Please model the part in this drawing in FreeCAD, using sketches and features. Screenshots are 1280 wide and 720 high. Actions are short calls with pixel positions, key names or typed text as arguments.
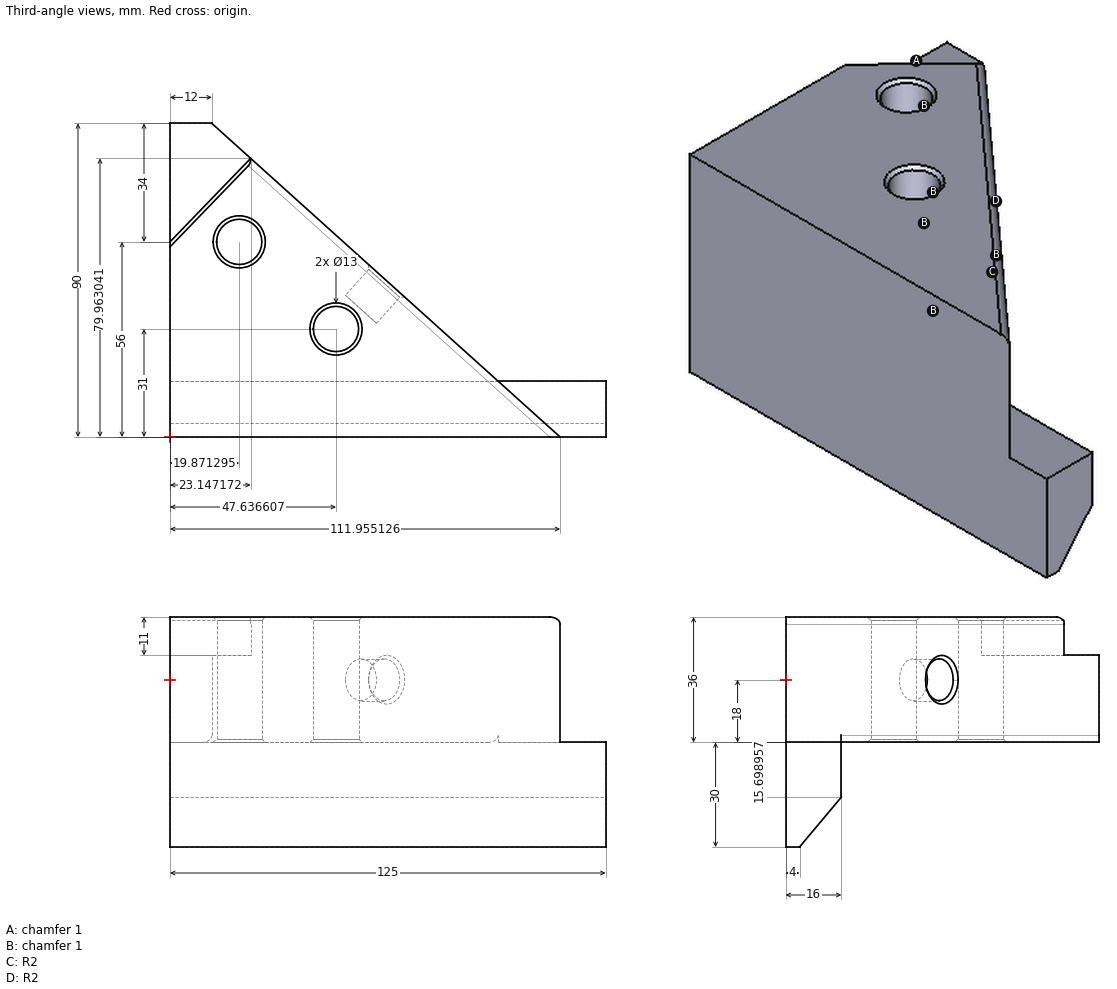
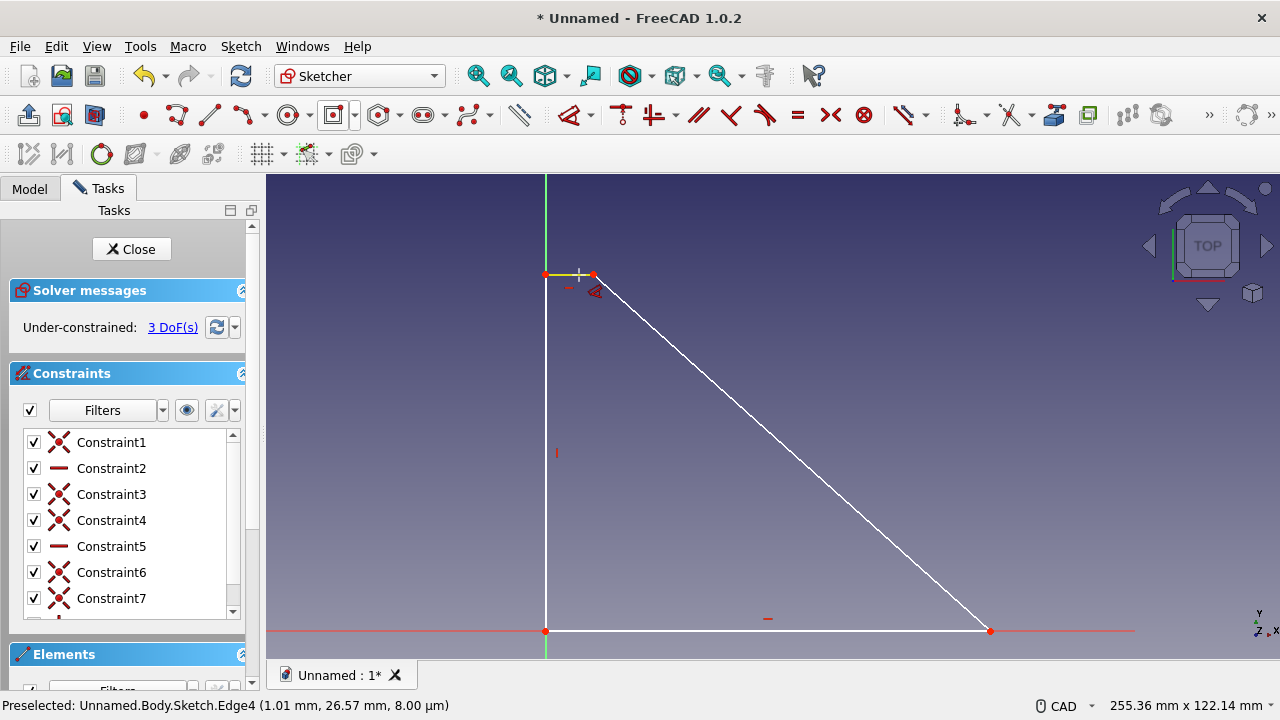
click(579, 275)
click(570, 241)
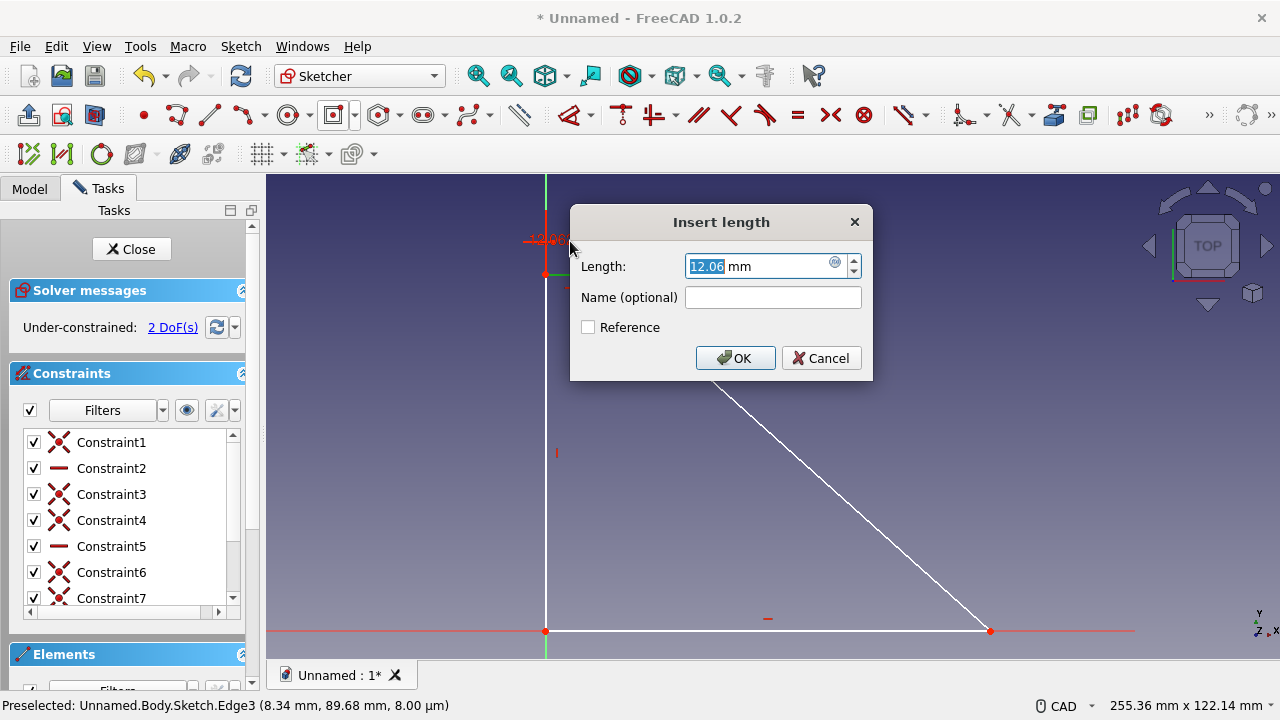
text(12)
key(Return)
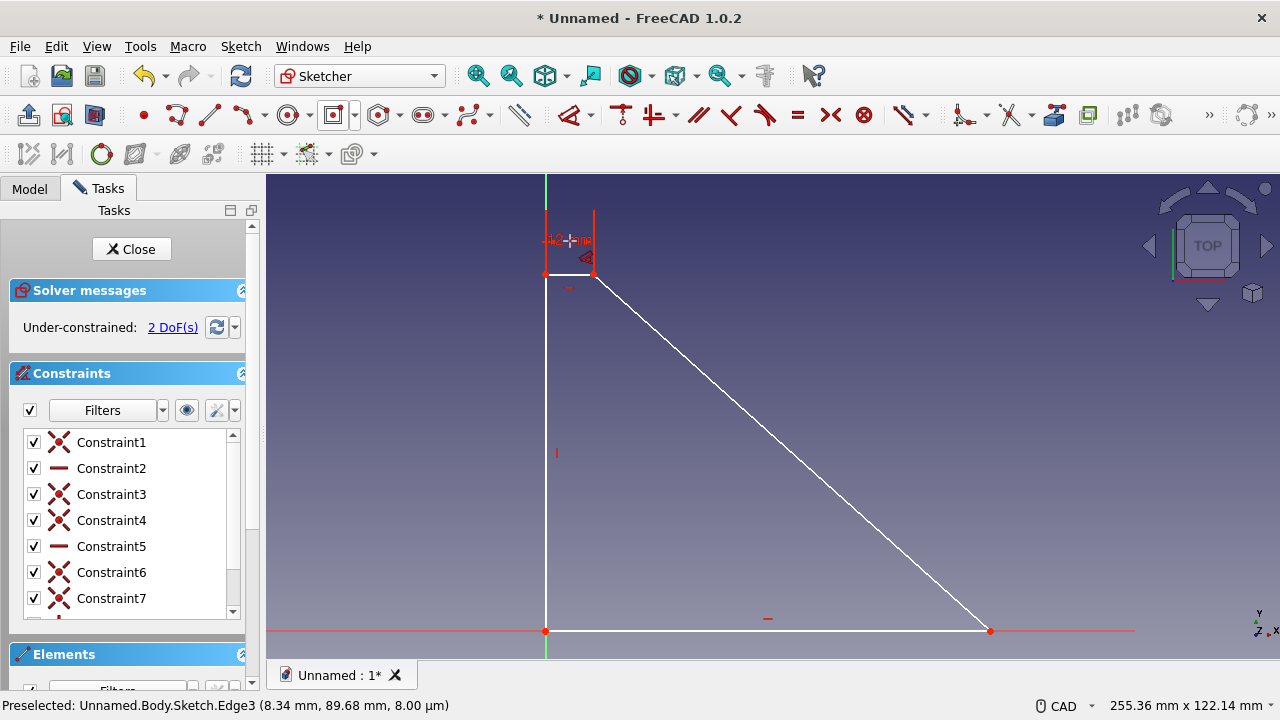
click(546, 382)
click(512, 453)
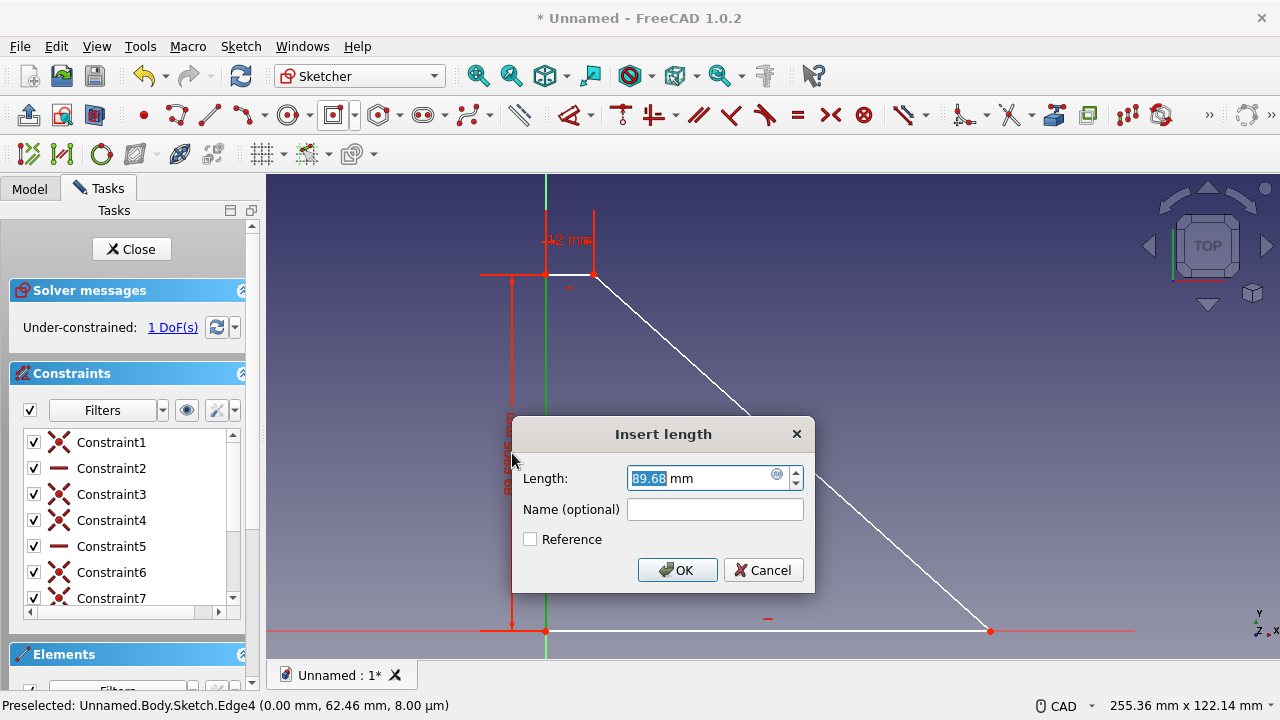
text(90)
key(Return)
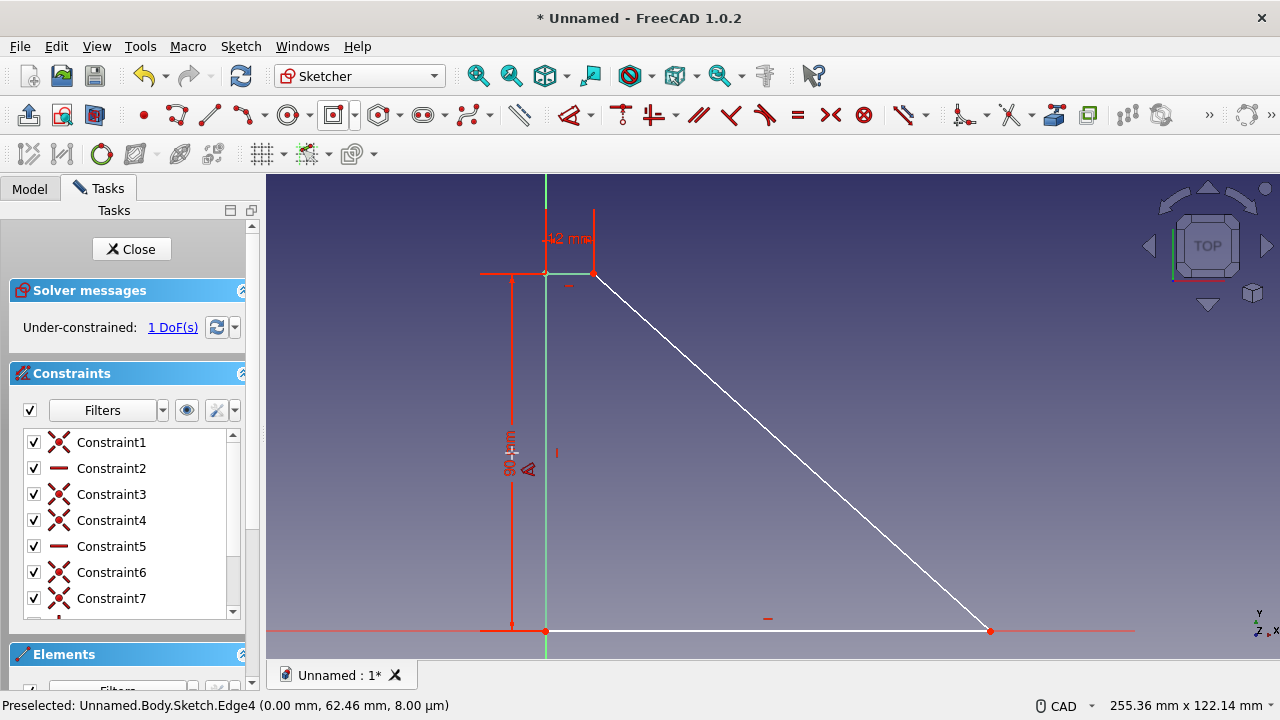
scroll(417, 255, down, 1)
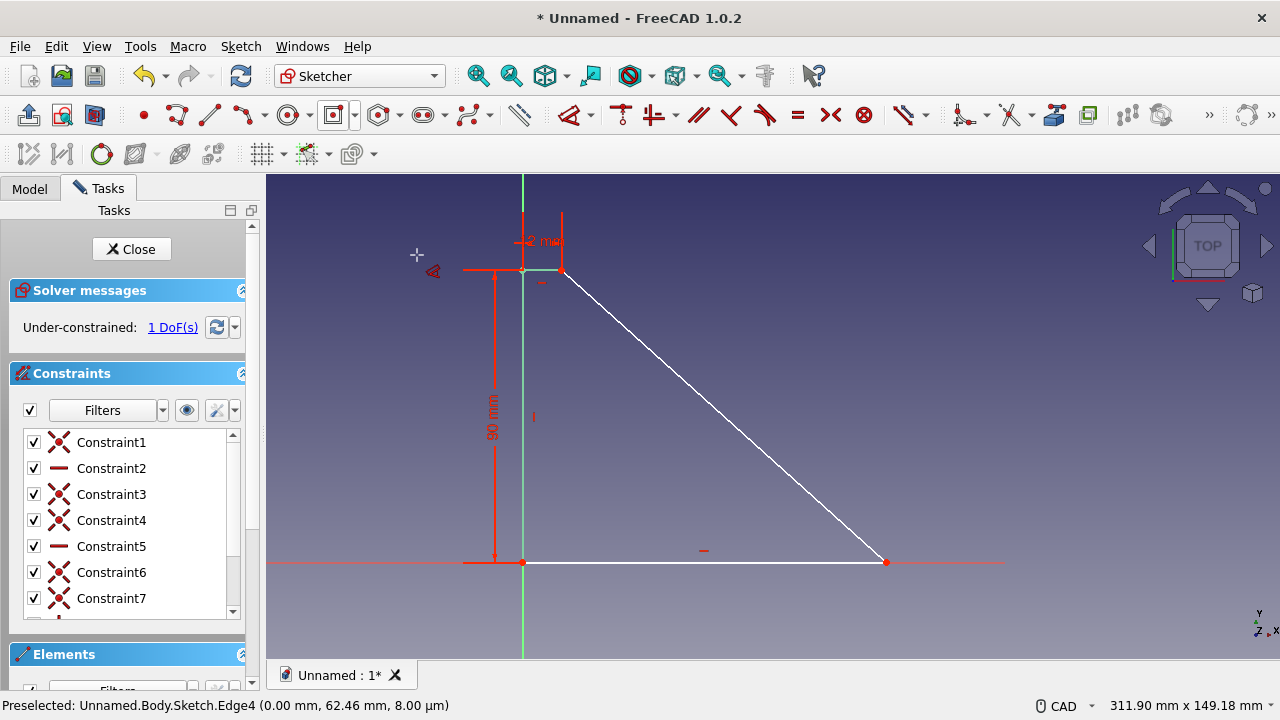
click(632, 563)
click(705, 597)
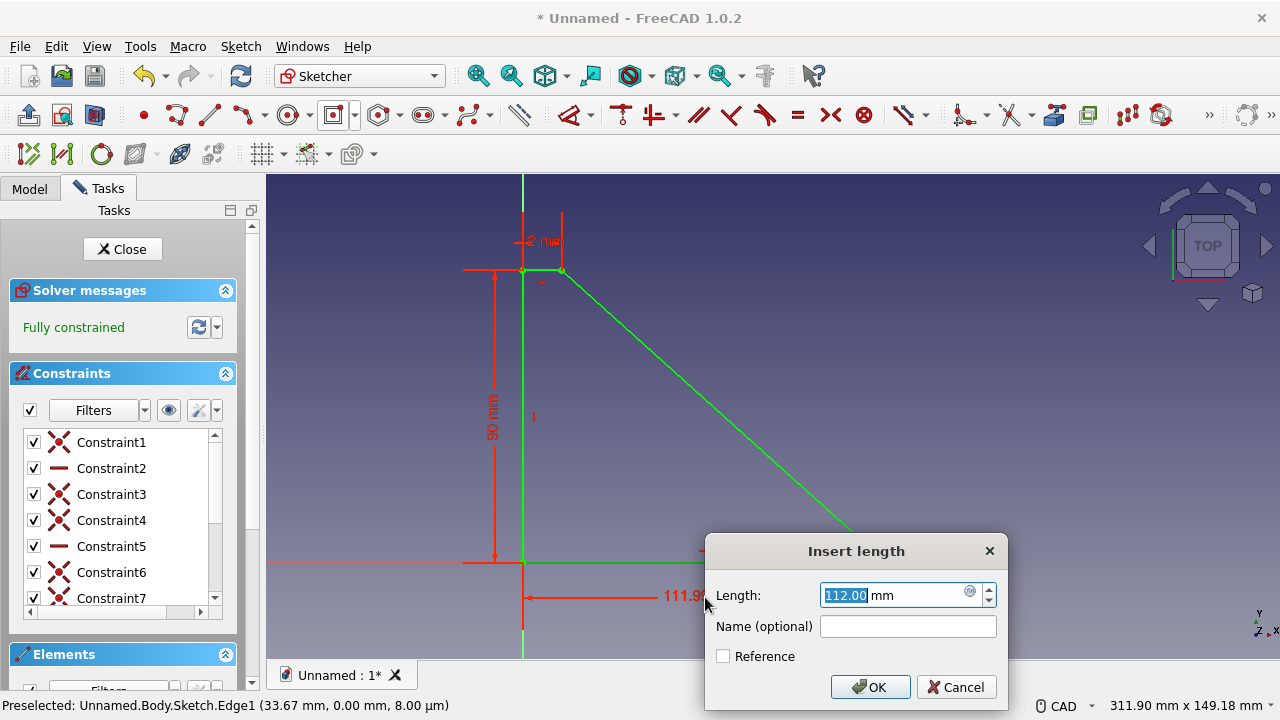
text(111.955126)
key(Return)
key(Escape)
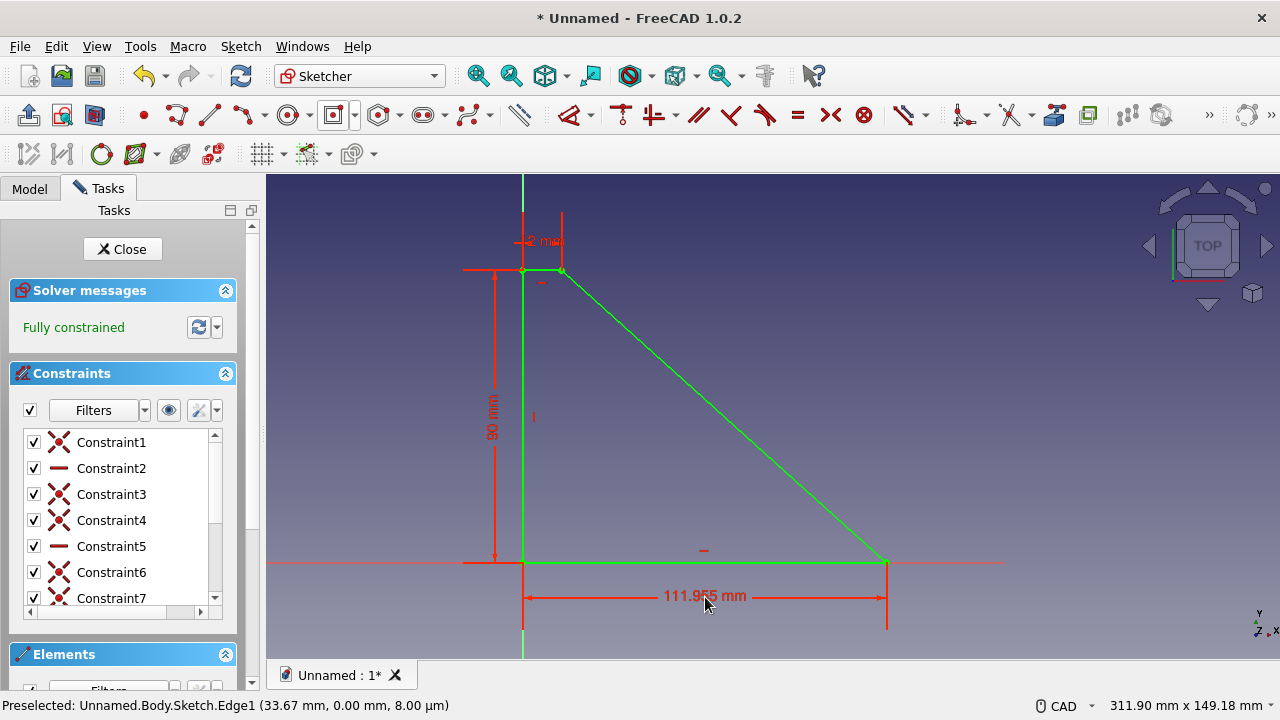
click(123, 249)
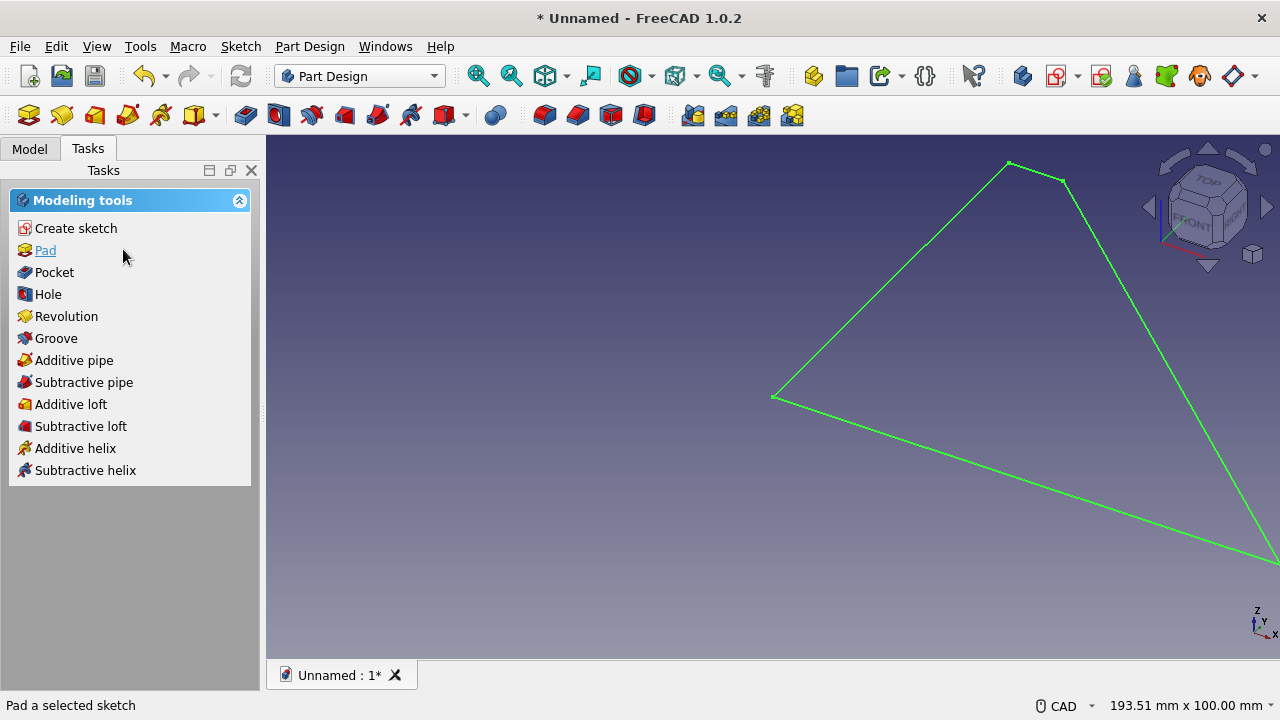
click(29, 116)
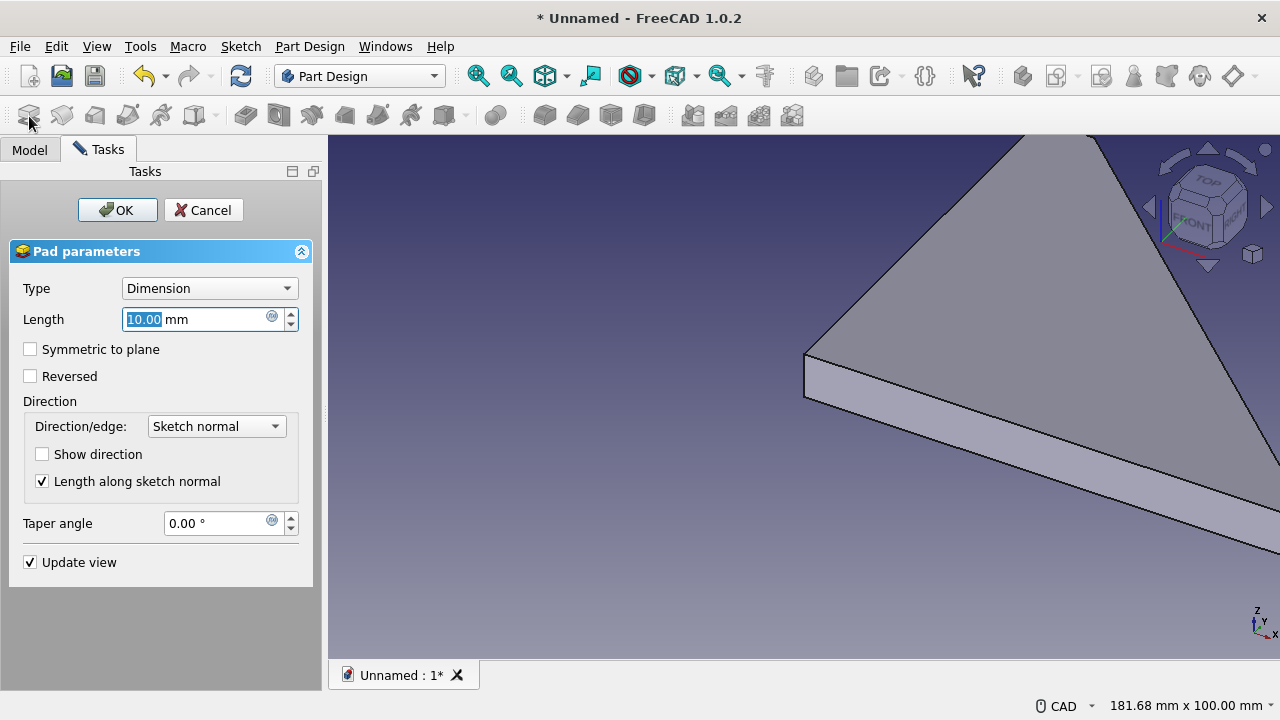
text(36)
key(Tab)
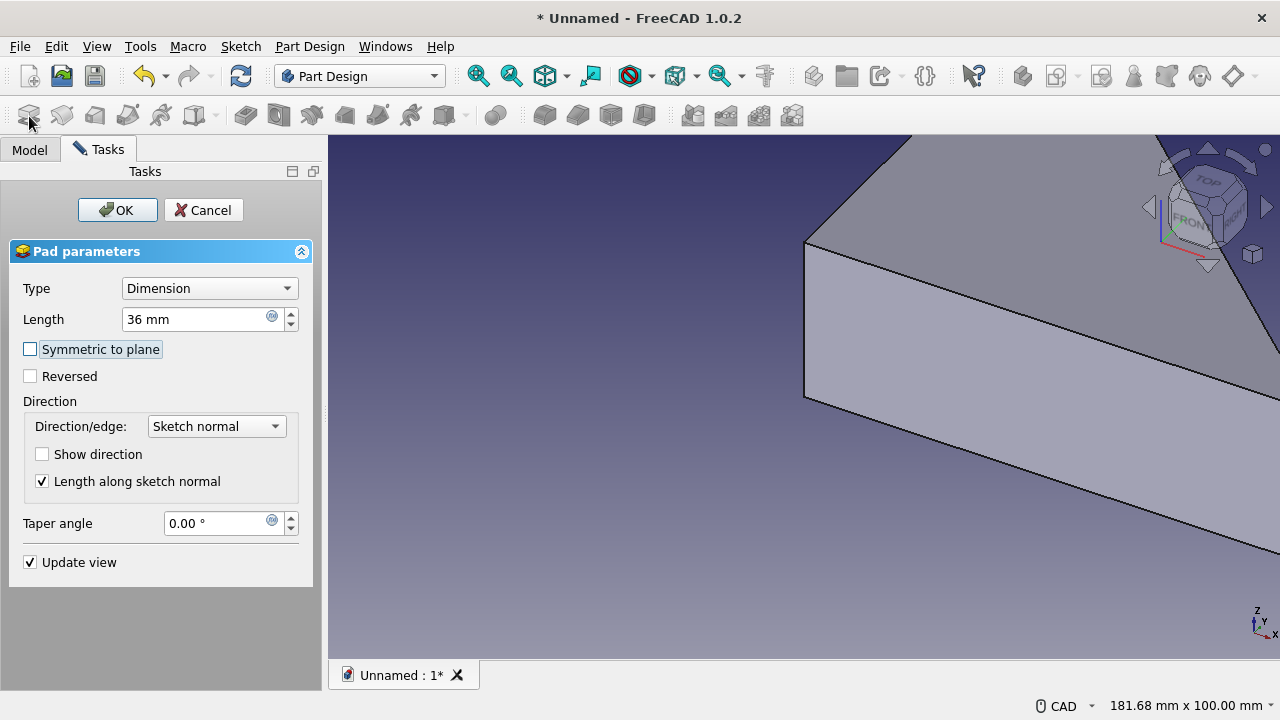
click(31, 349)